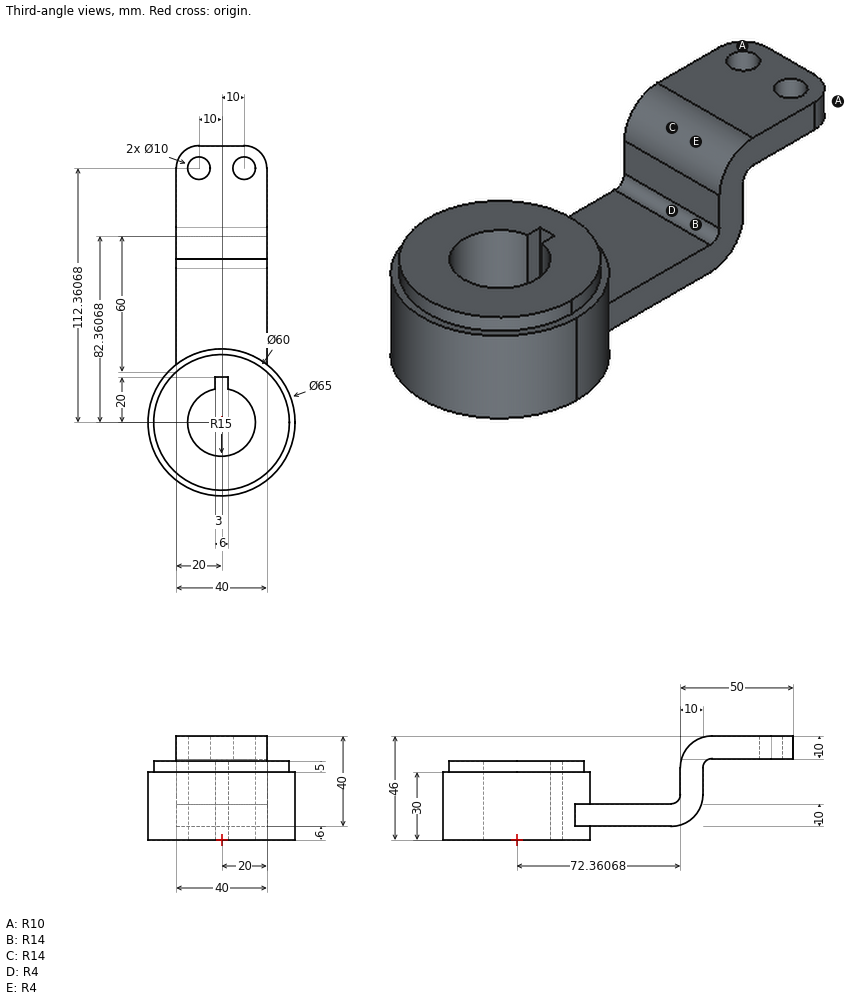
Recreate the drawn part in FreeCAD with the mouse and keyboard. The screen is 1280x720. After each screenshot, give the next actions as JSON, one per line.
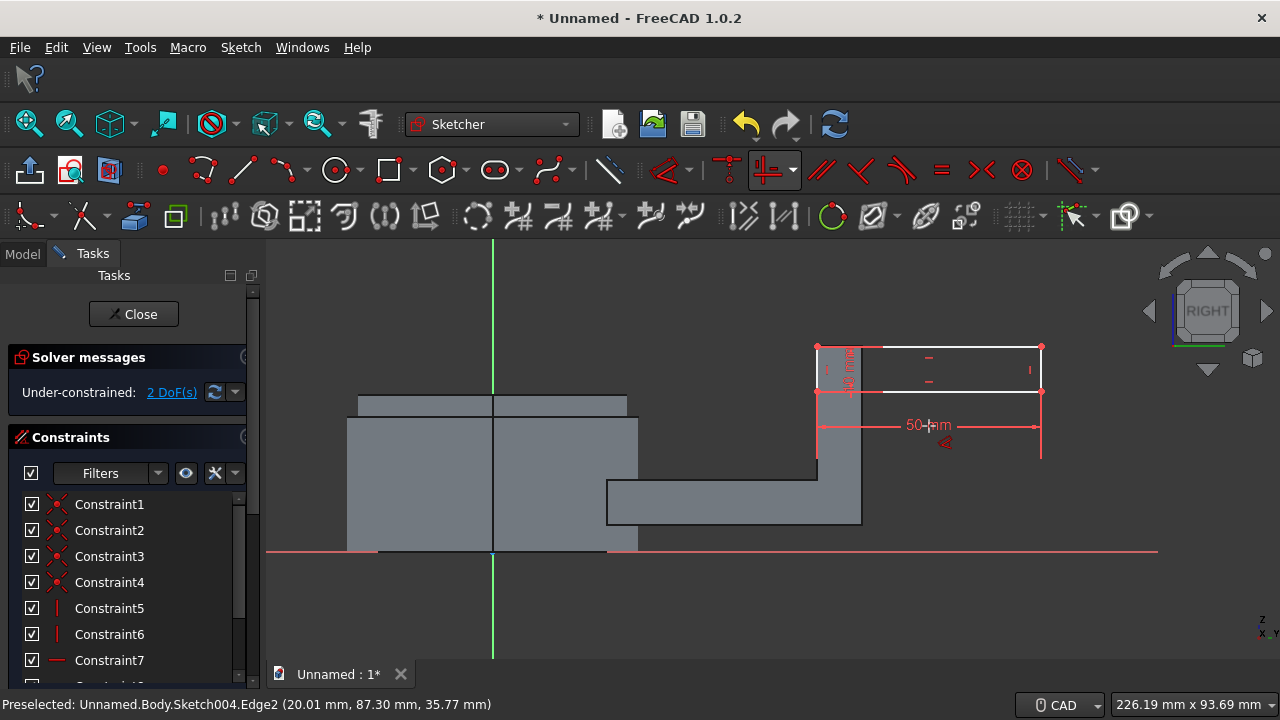
{"action": "left_click", "coordinate": [817, 347]}
{"action": "left_click", "coordinate": [459, 449]}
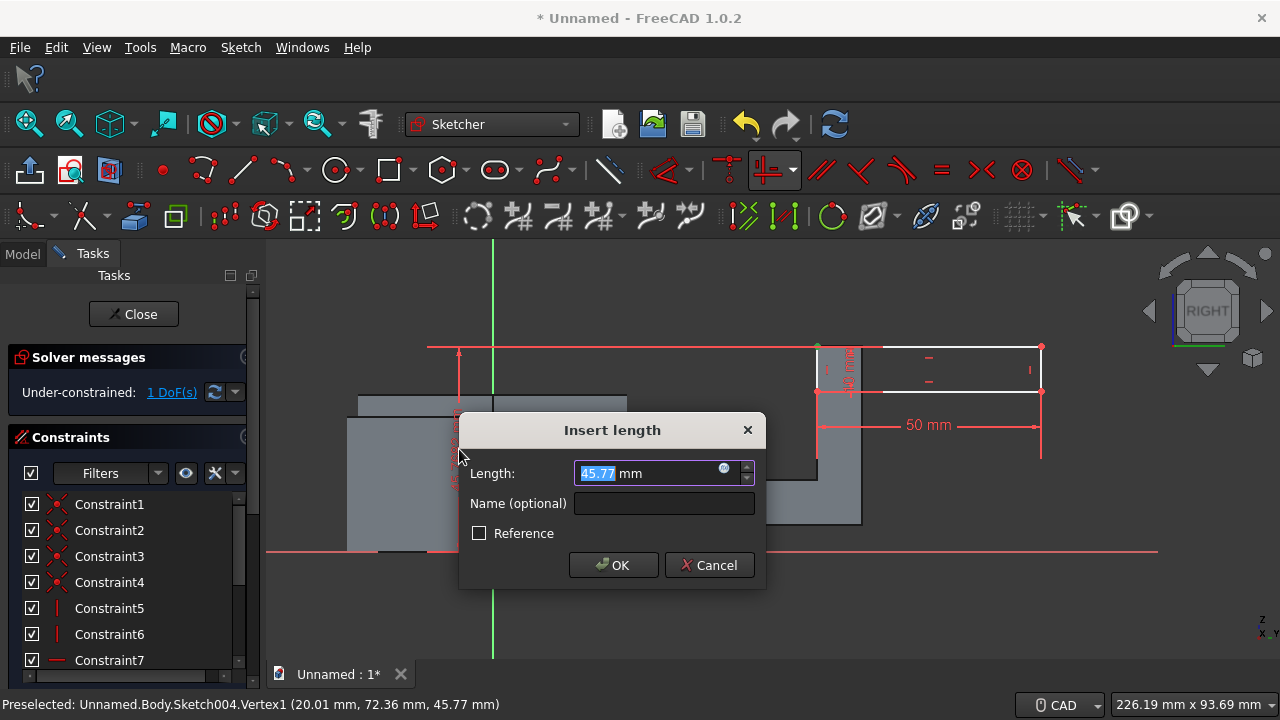
{"action": "type", "text": "46"}
{"action": "key", "text": "Return"}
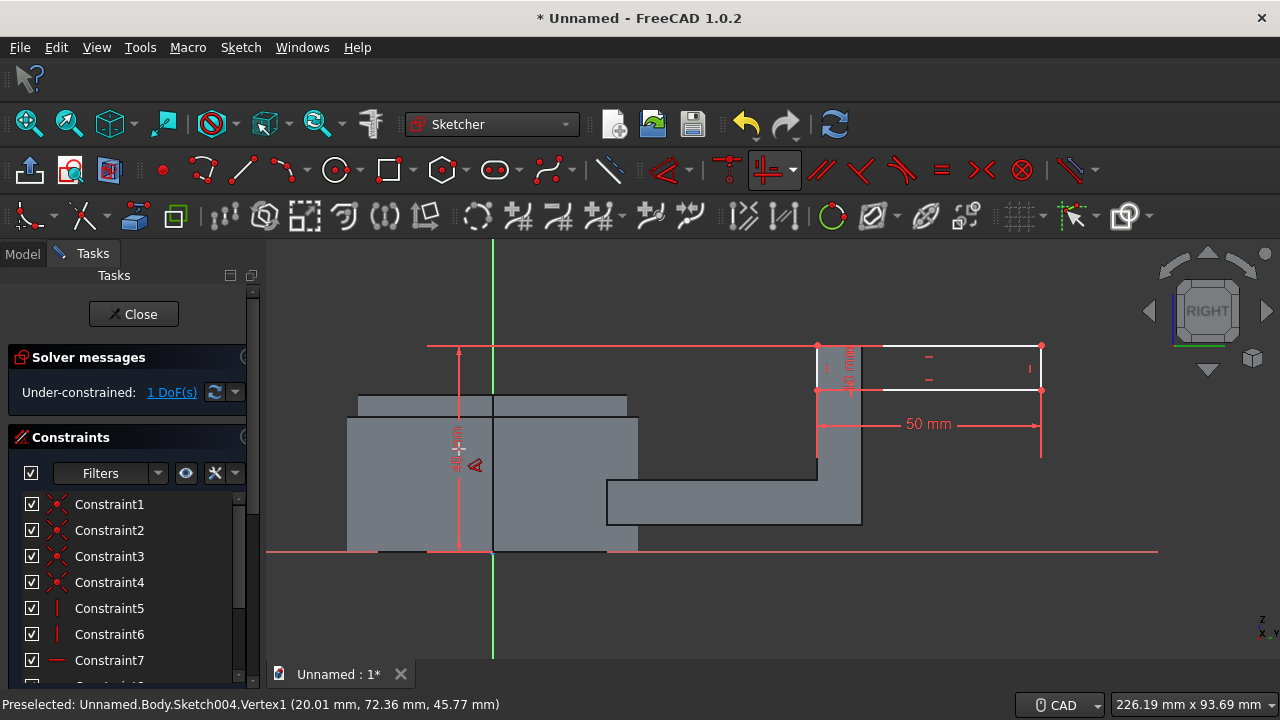
{"action": "left_click", "coordinate": [817, 346]}
{"action": "left_click", "coordinate": [655, 586]}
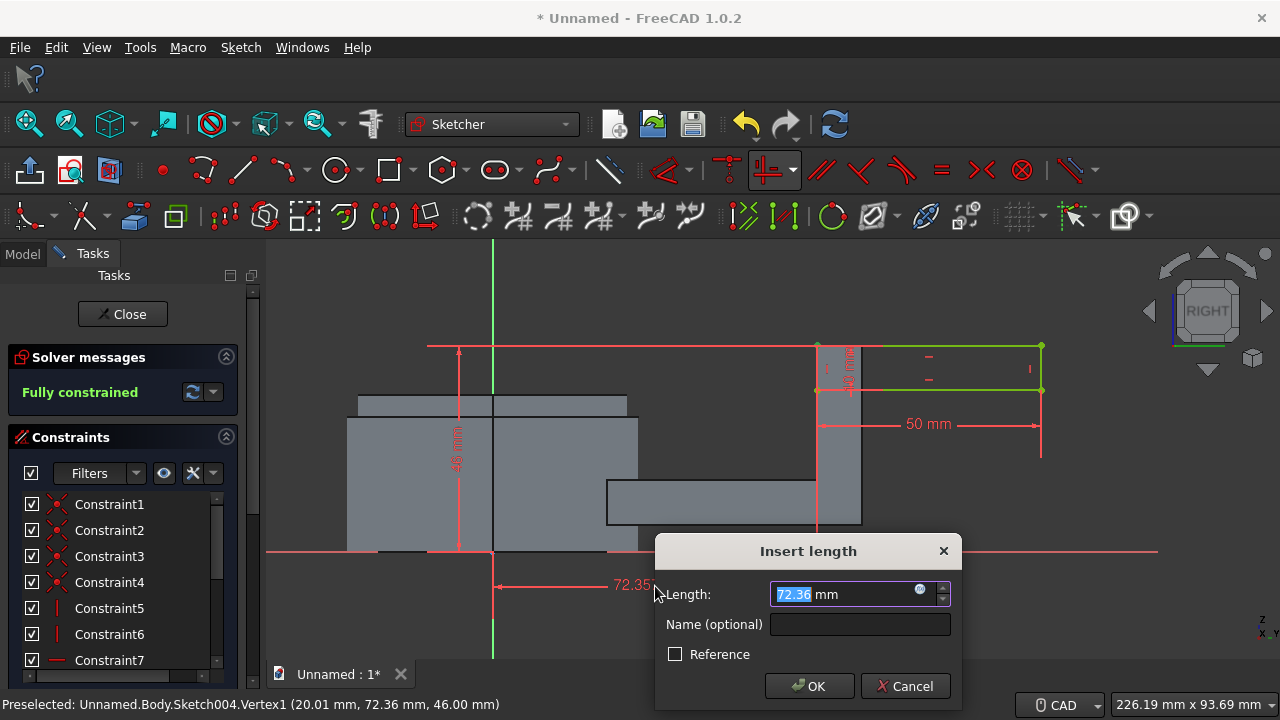
{"action": "type", "text": "72.36068"}
{"action": "key", "text": "Return"}
{"action": "key", "text": "Escape"}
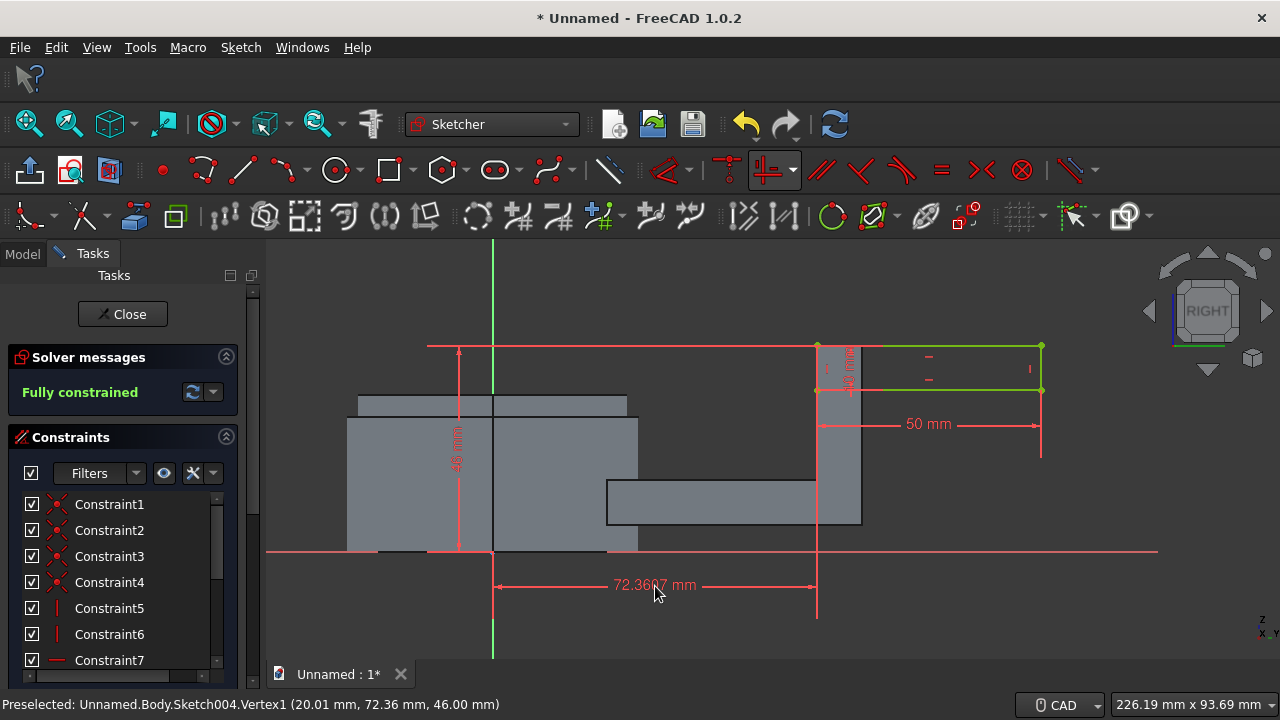
{"action": "left_click", "coordinate": [123, 314]}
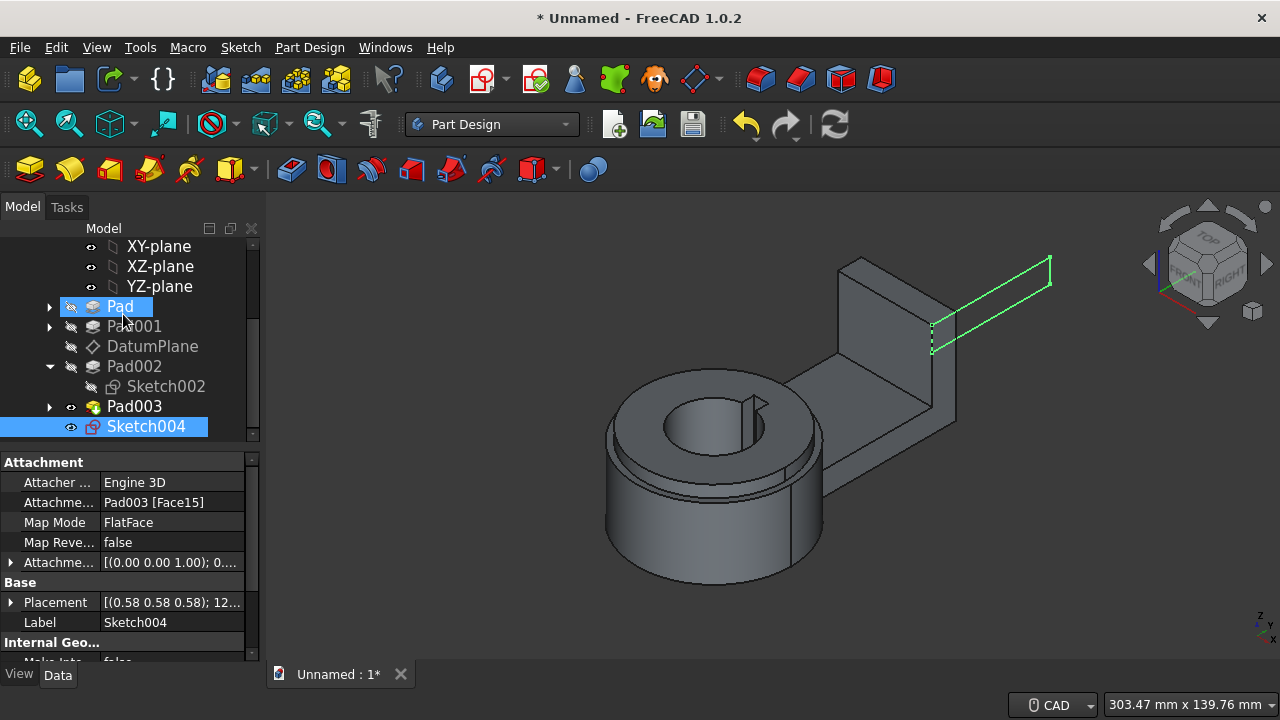
{"action": "left_click", "coordinate": [30, 170]}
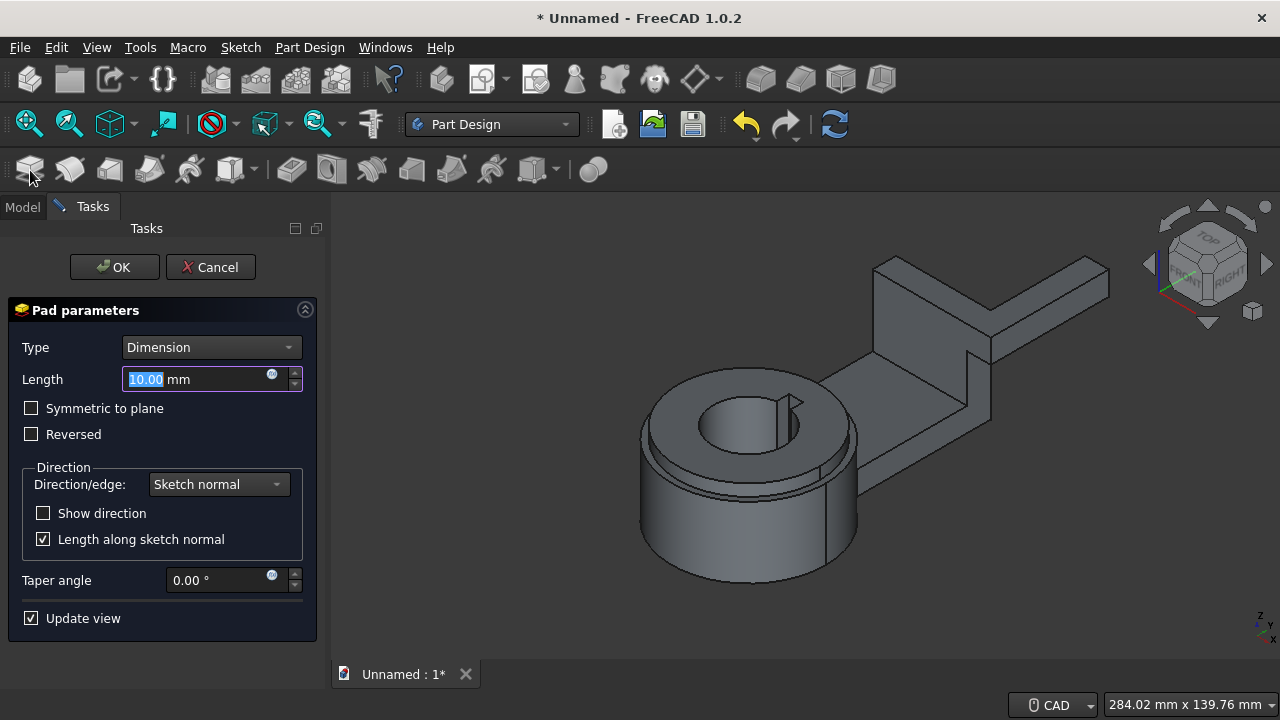
{"action": "type", "text": "40"}
{"action": "key", "text": "Tab"}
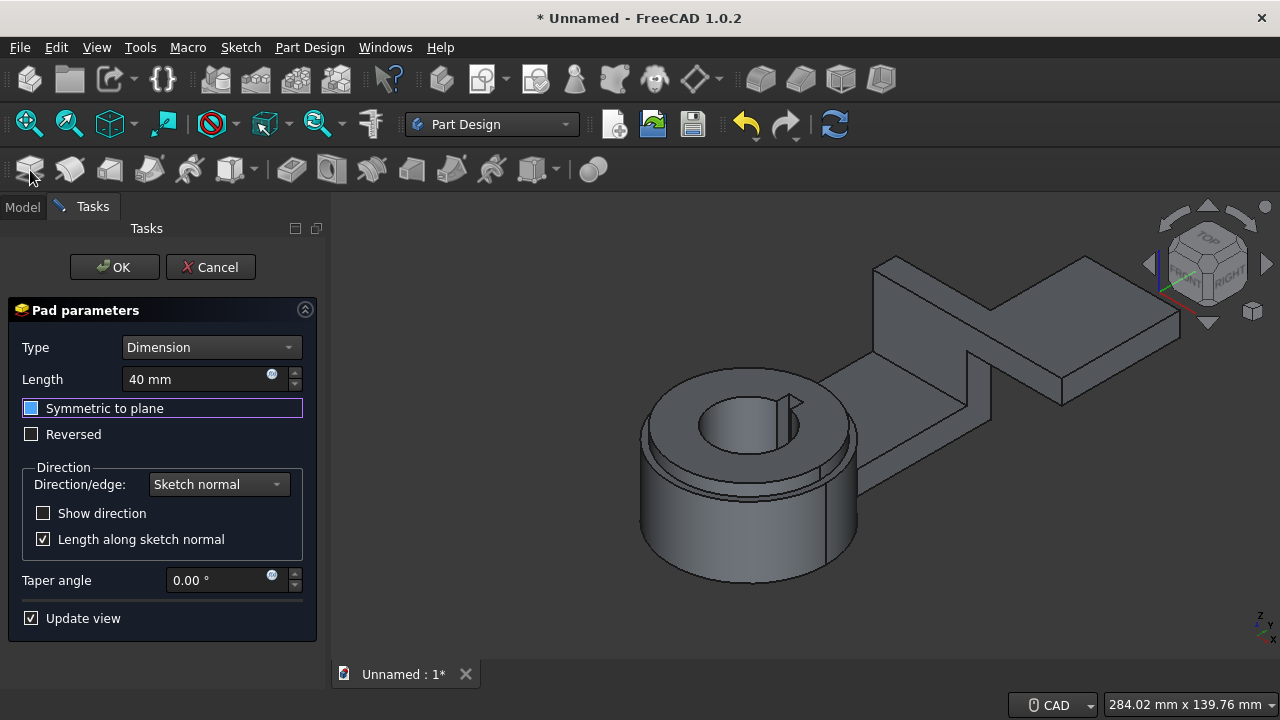
{"action": "left_click", "coordinate": [30, 434]}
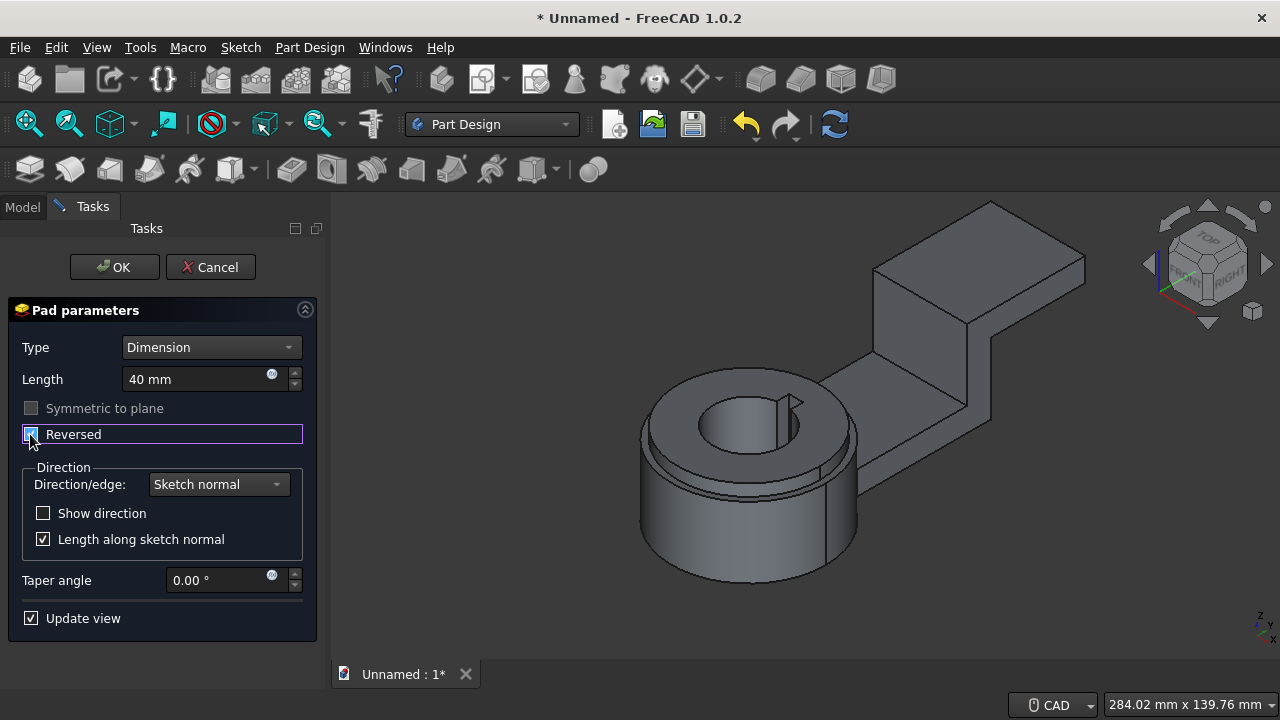
{"action": "left_click", "coordinate": [115, 267]}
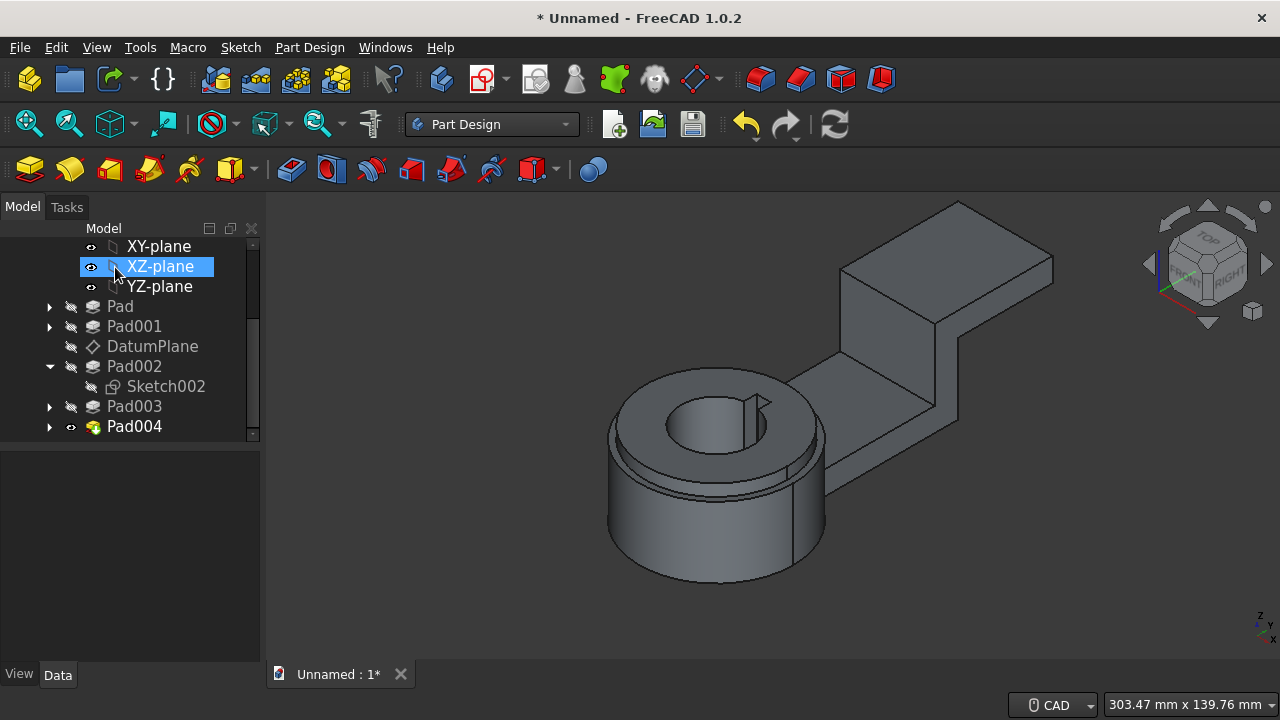
{"action": "left_click", "coordinate": [30, 124]}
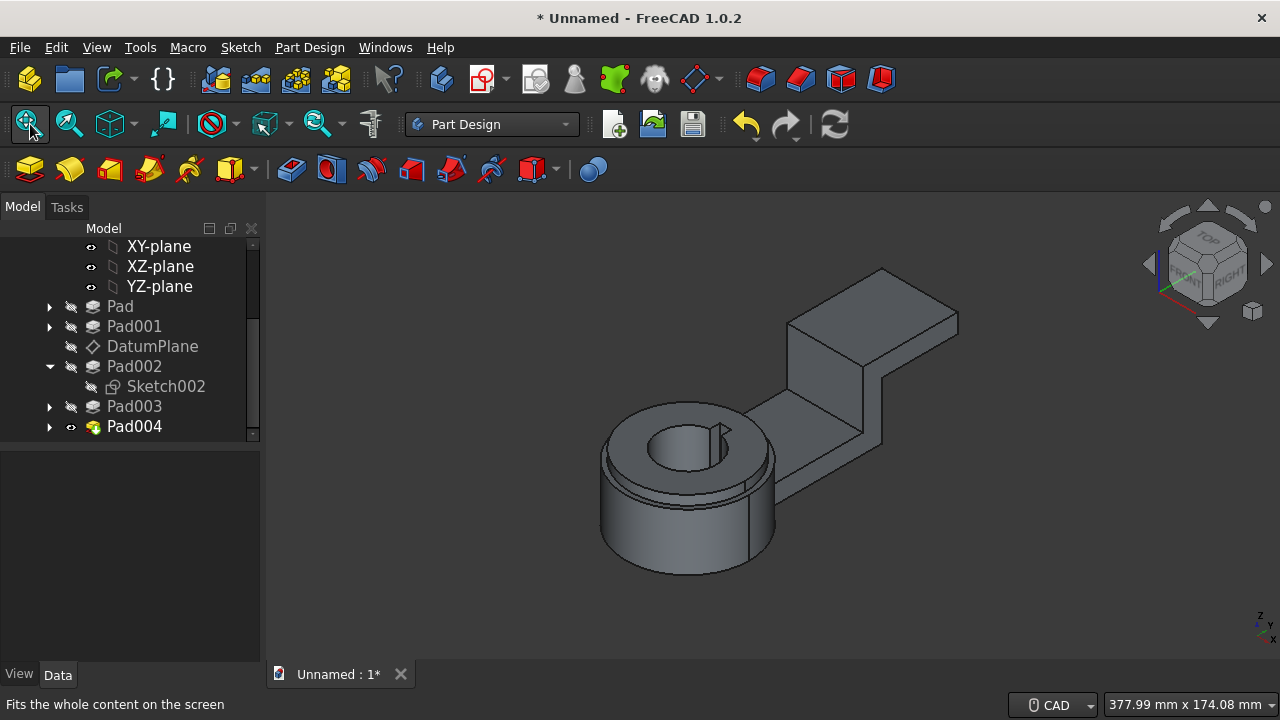
{"action": "key", "text": "2"}